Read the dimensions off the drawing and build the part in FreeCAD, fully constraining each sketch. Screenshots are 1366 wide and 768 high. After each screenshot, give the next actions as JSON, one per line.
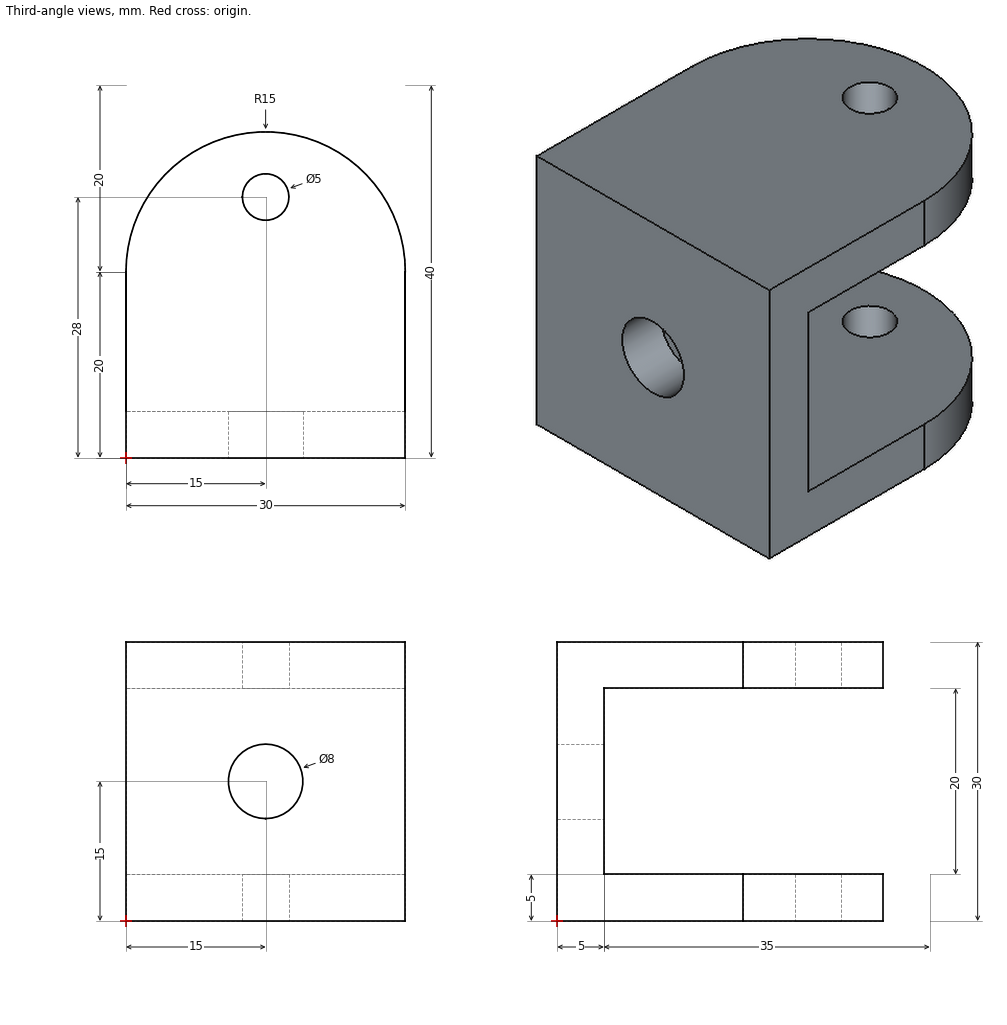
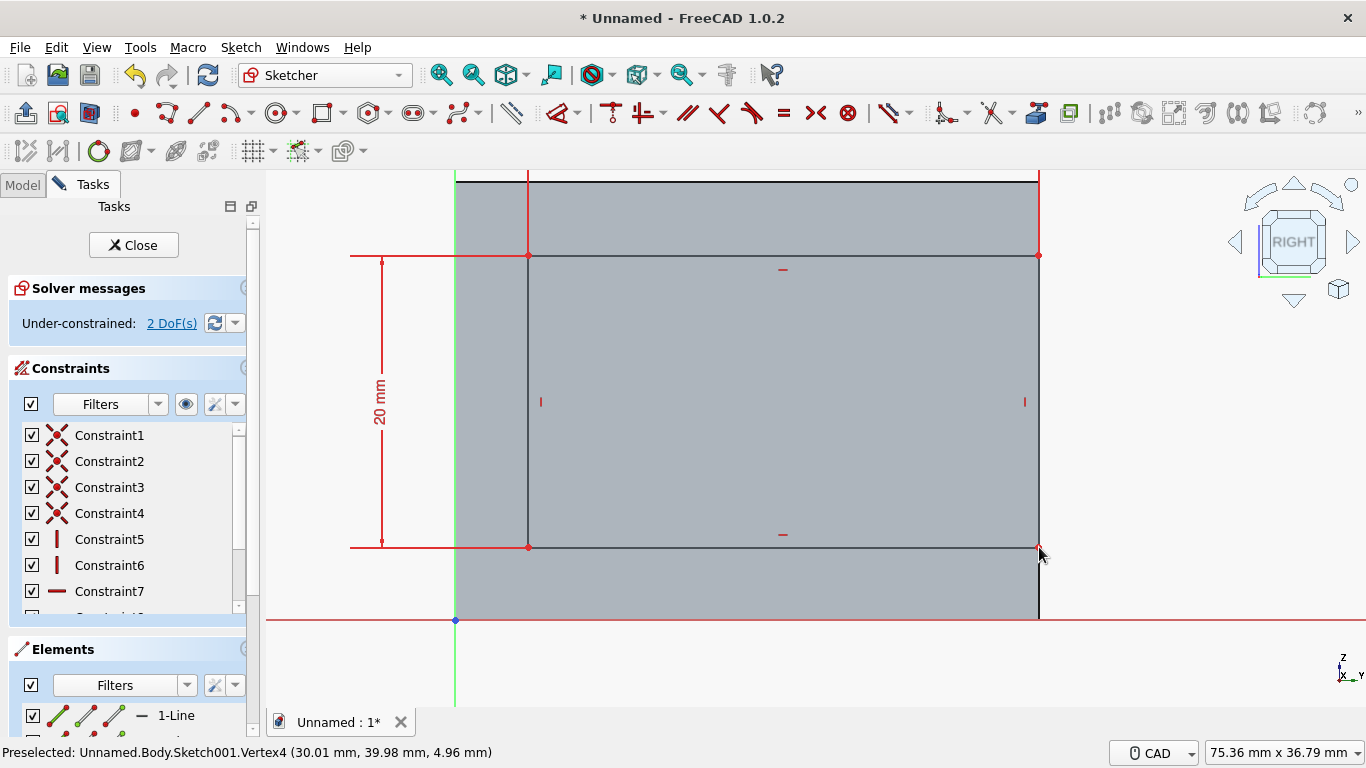
{"action": "left_click", "coordinate": [528, 256]}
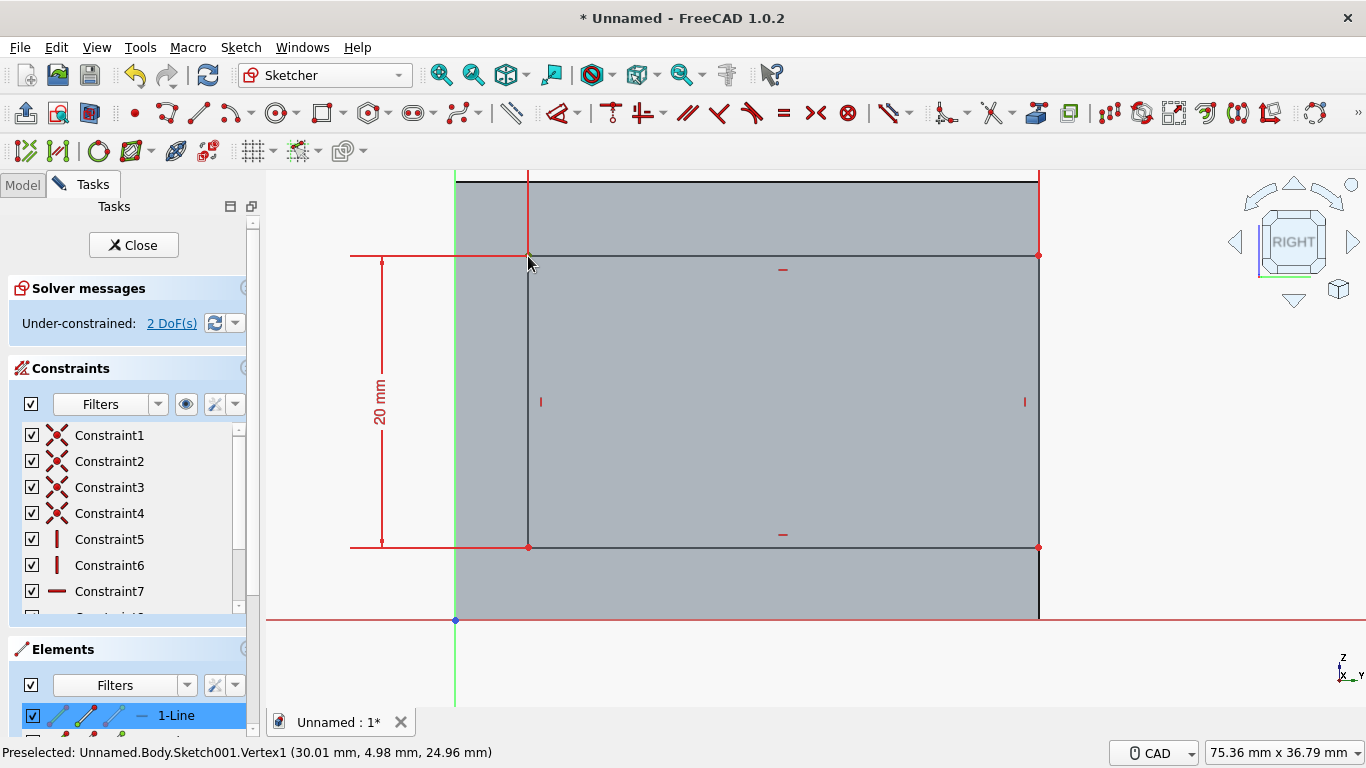
{"action": "left_click", "coordinate": [580, 114]}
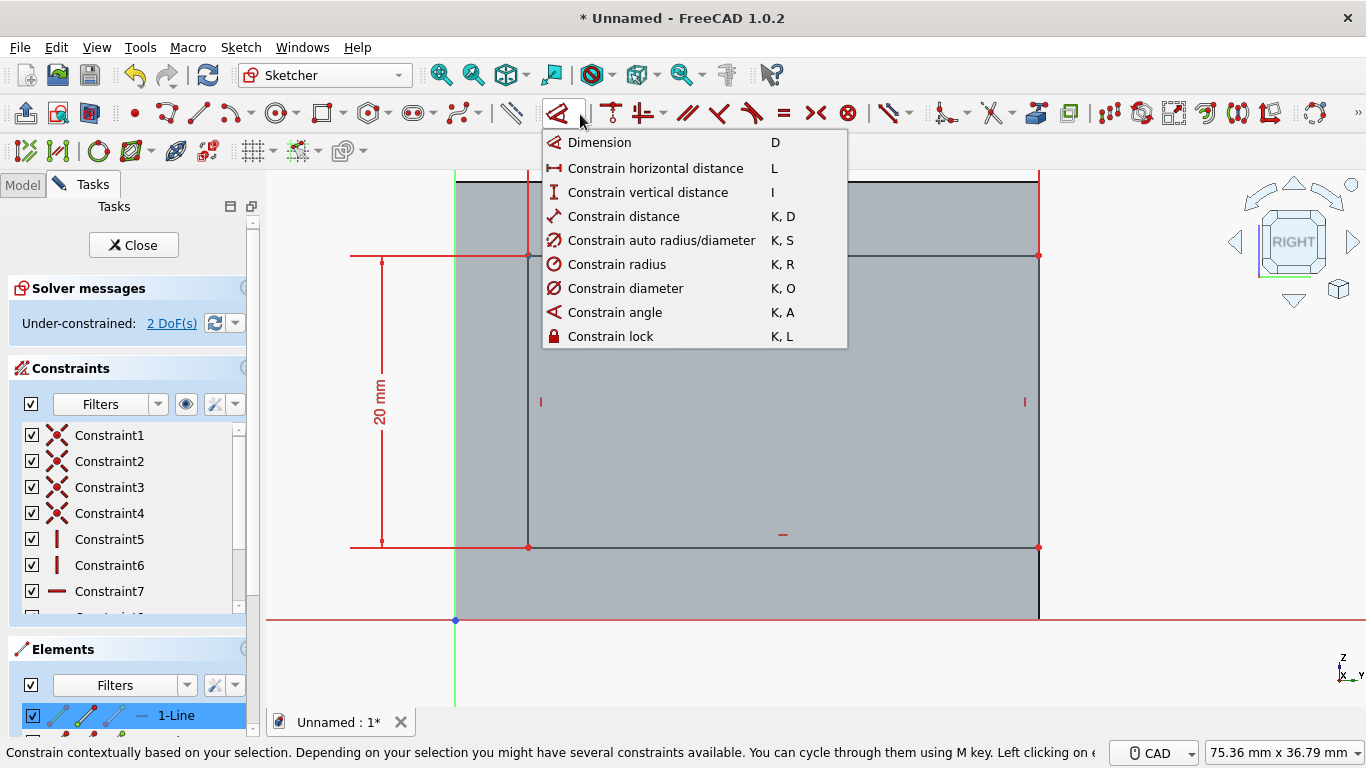
{"action": "left_click", "coordinate": [695, 168]}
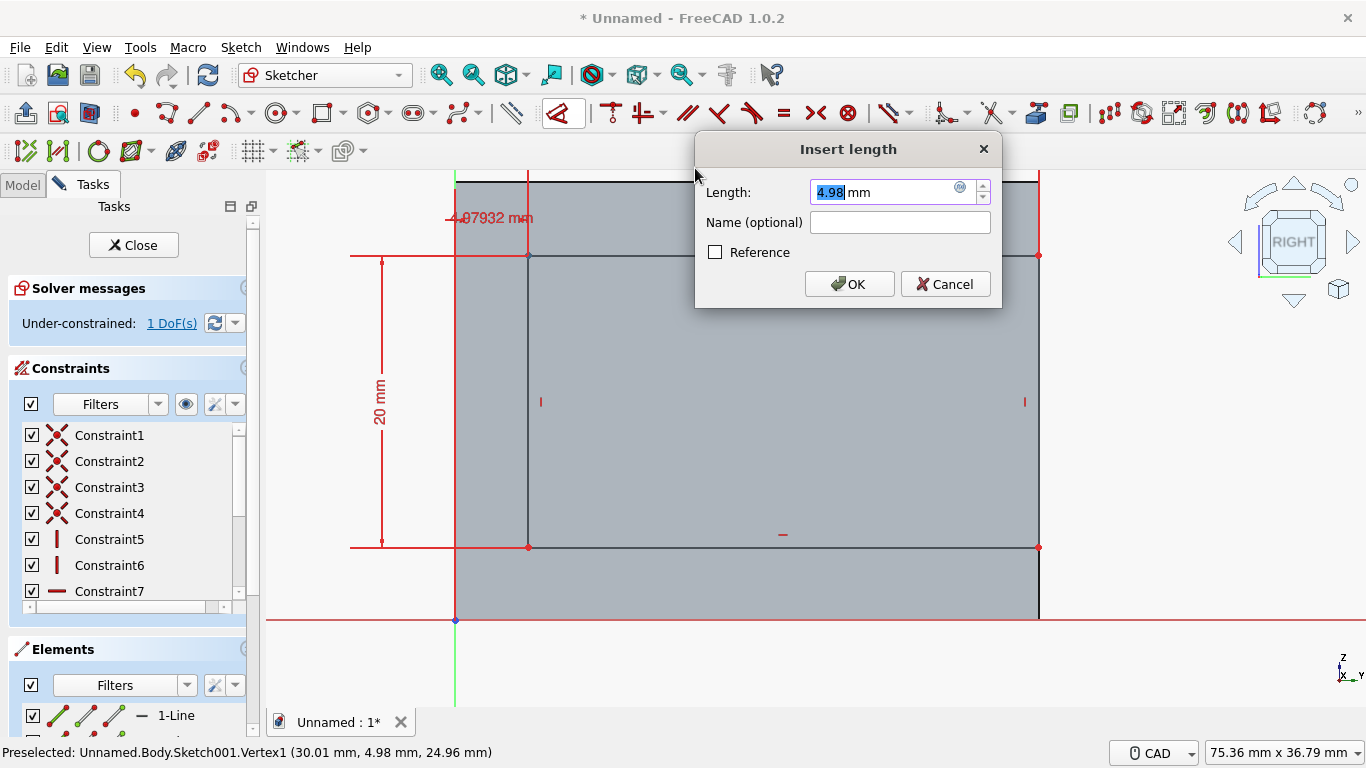
{"action": "type", "text": "5"}
{"action": "key", "text": "Return"}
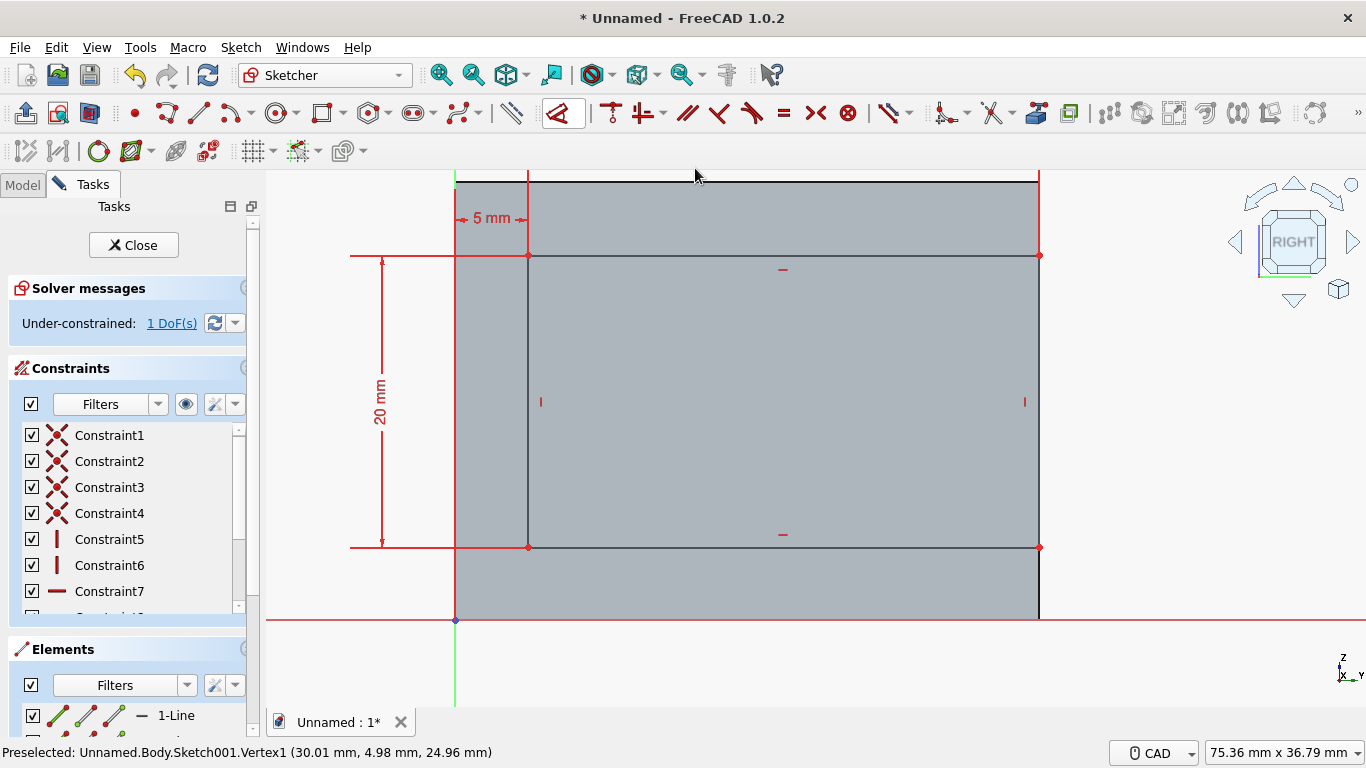
{"action": "left_click", "coordinate": [528, 548]}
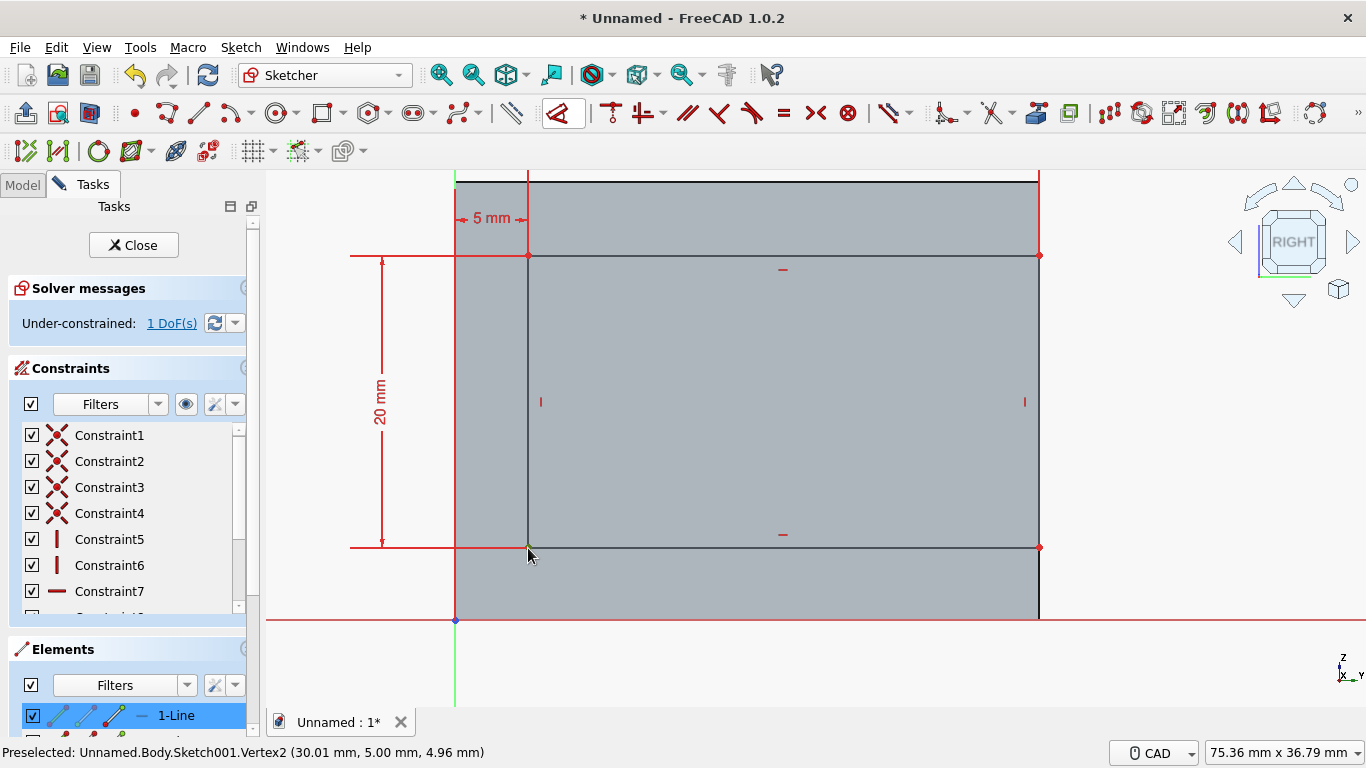
{"action": "left_click", "coordinate": [580, 114]}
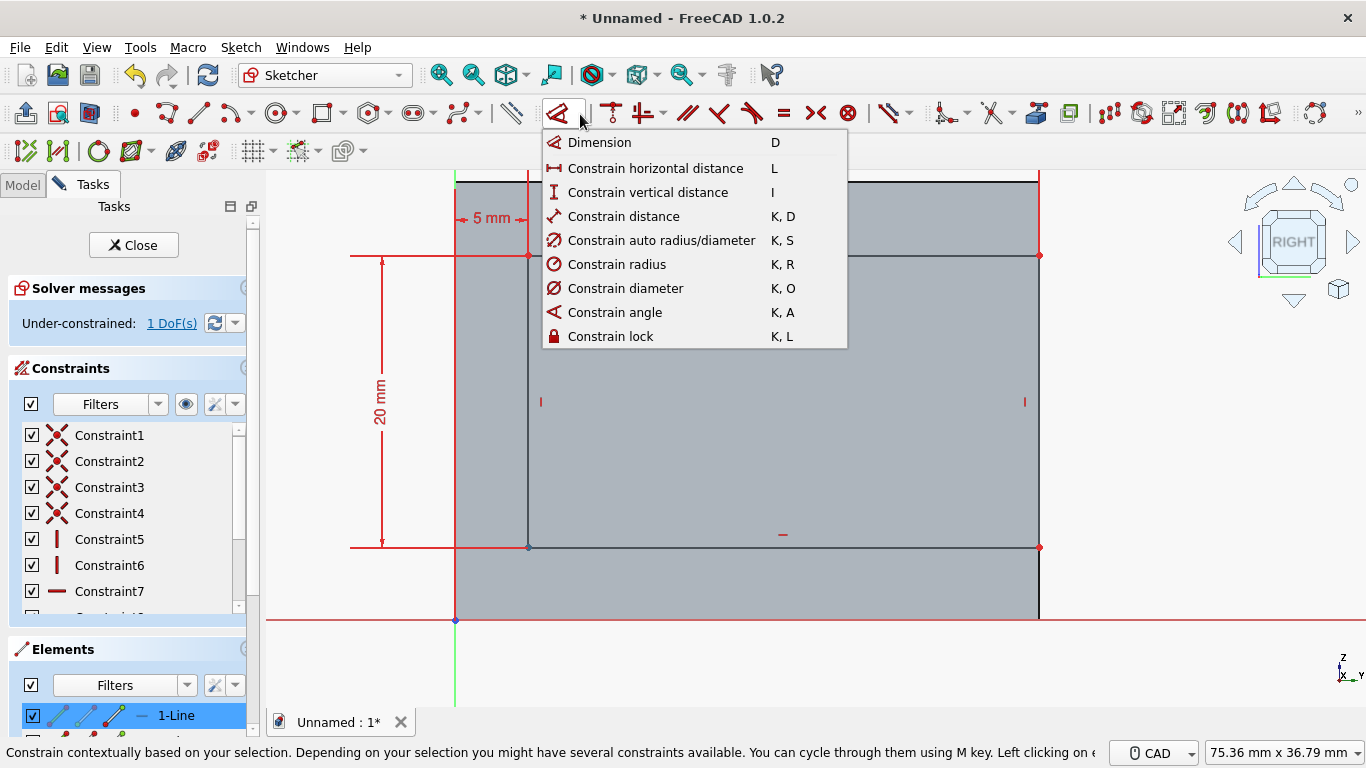
{"action": "left_click", "coordinate": [695, 192]}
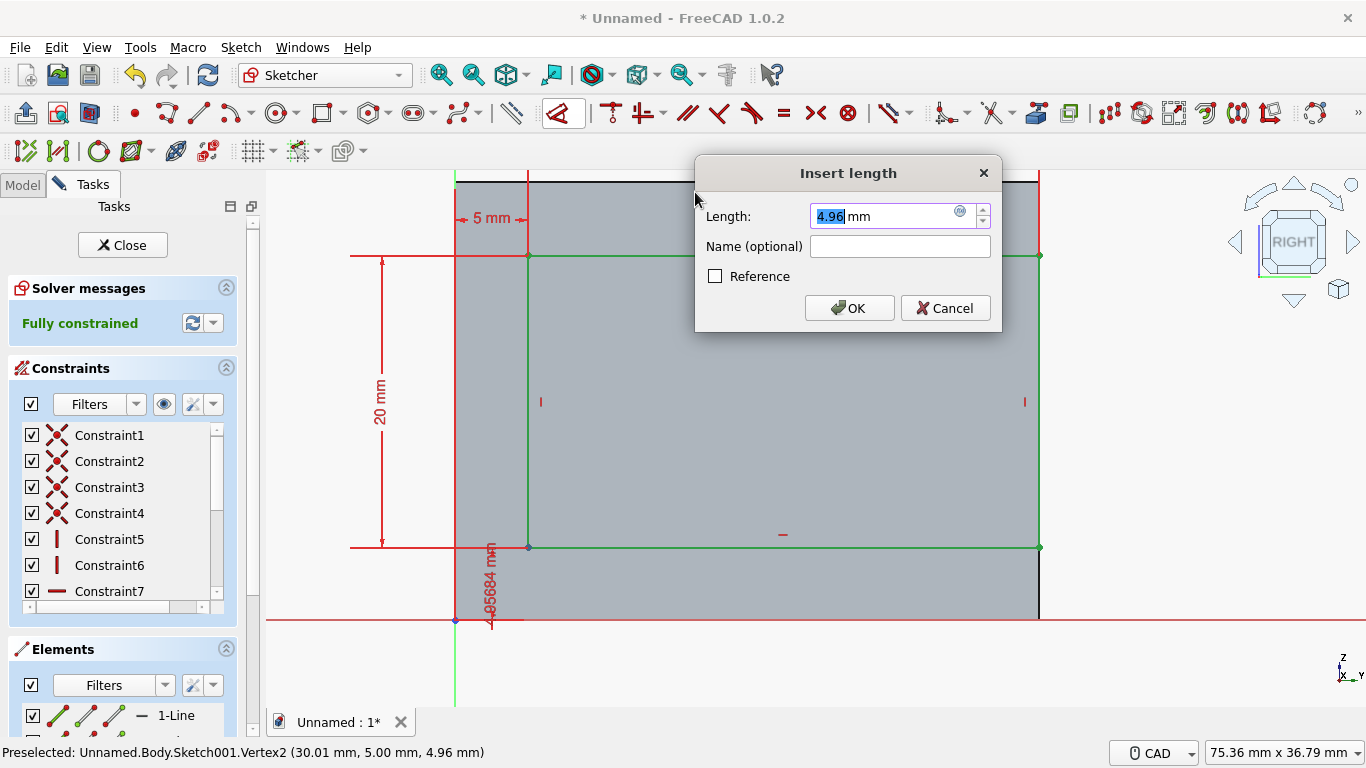
{"action": "type", "text": "5"}
{"action": "key", "text": "Return"}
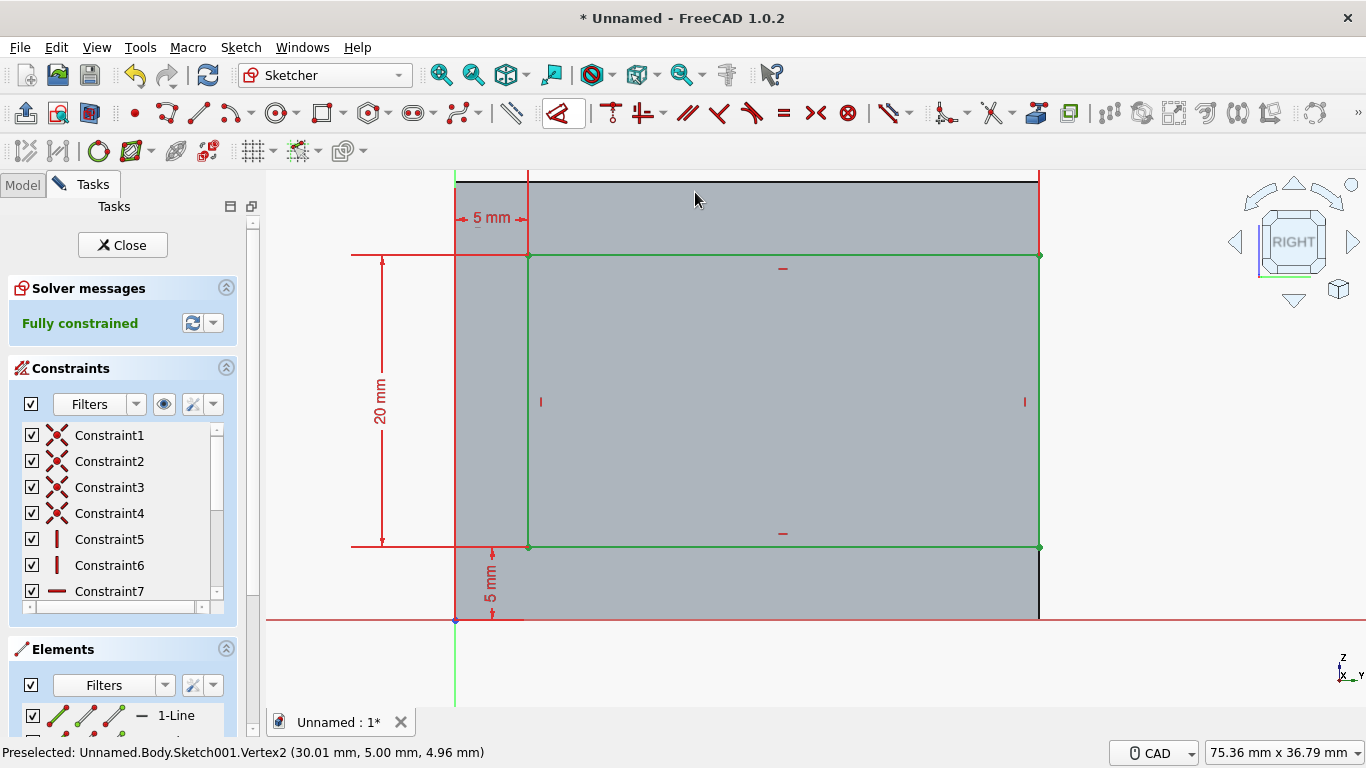
{"action": "left_click", "coordinate": [123, 245]}